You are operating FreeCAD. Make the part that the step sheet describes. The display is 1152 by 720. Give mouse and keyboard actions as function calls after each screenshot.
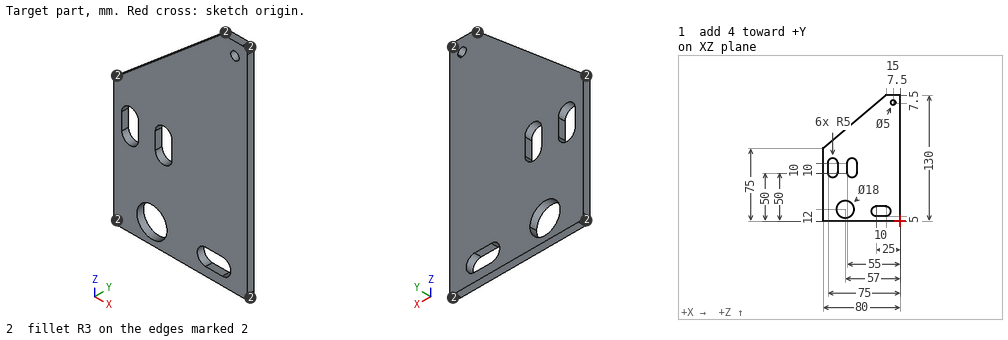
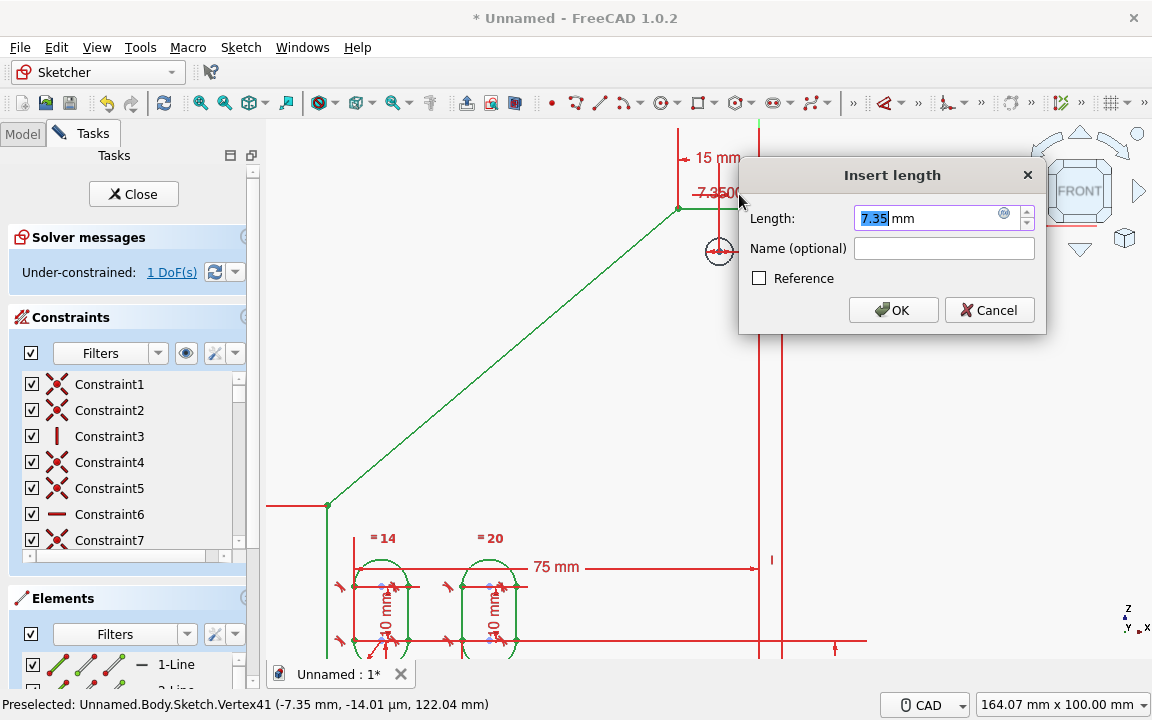
text(7.5)
key(Return)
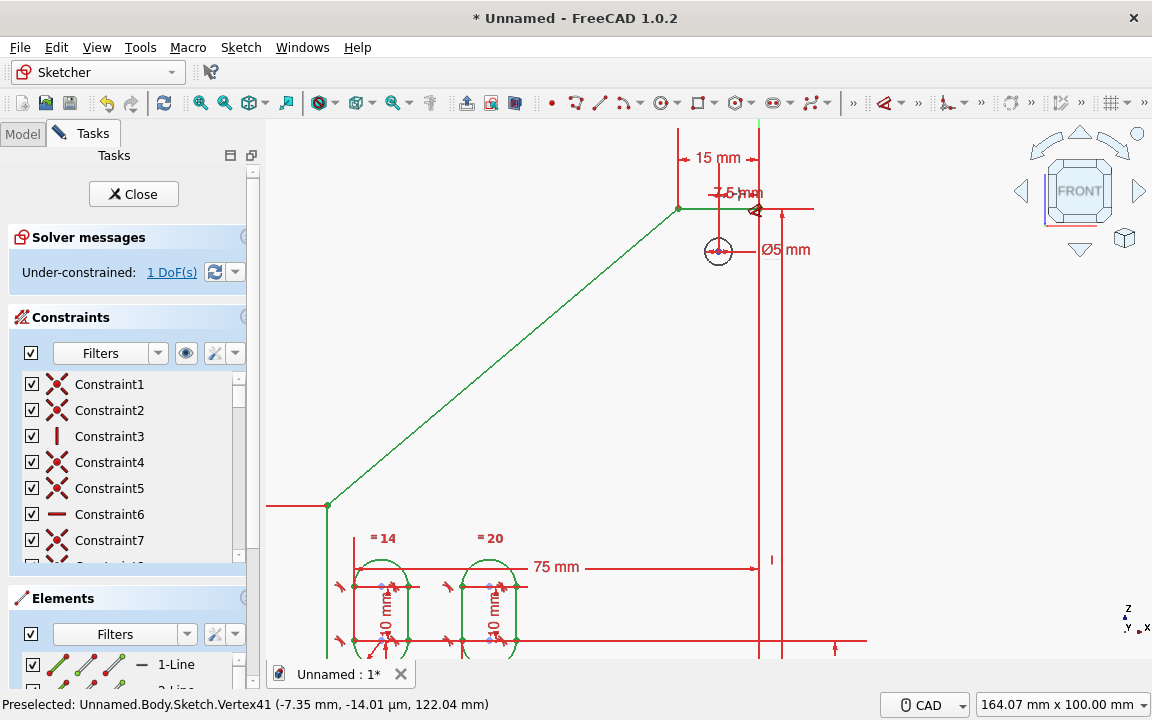
click(678, 209)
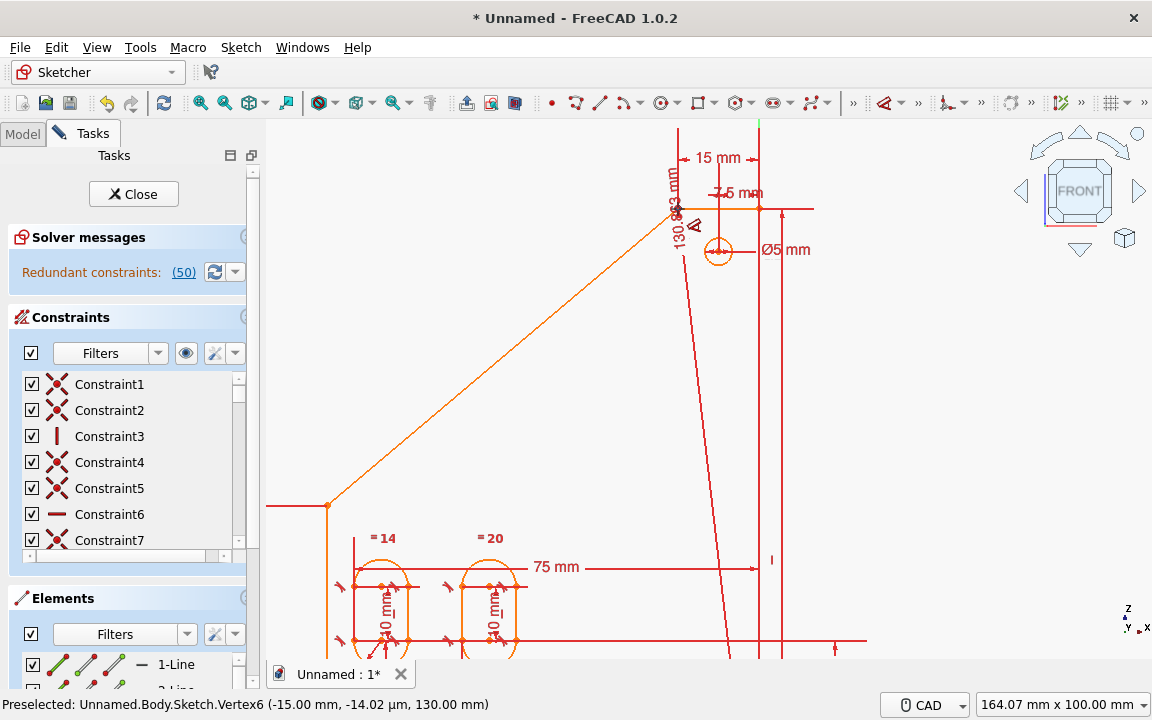
click(719, 252)
click(644, 220)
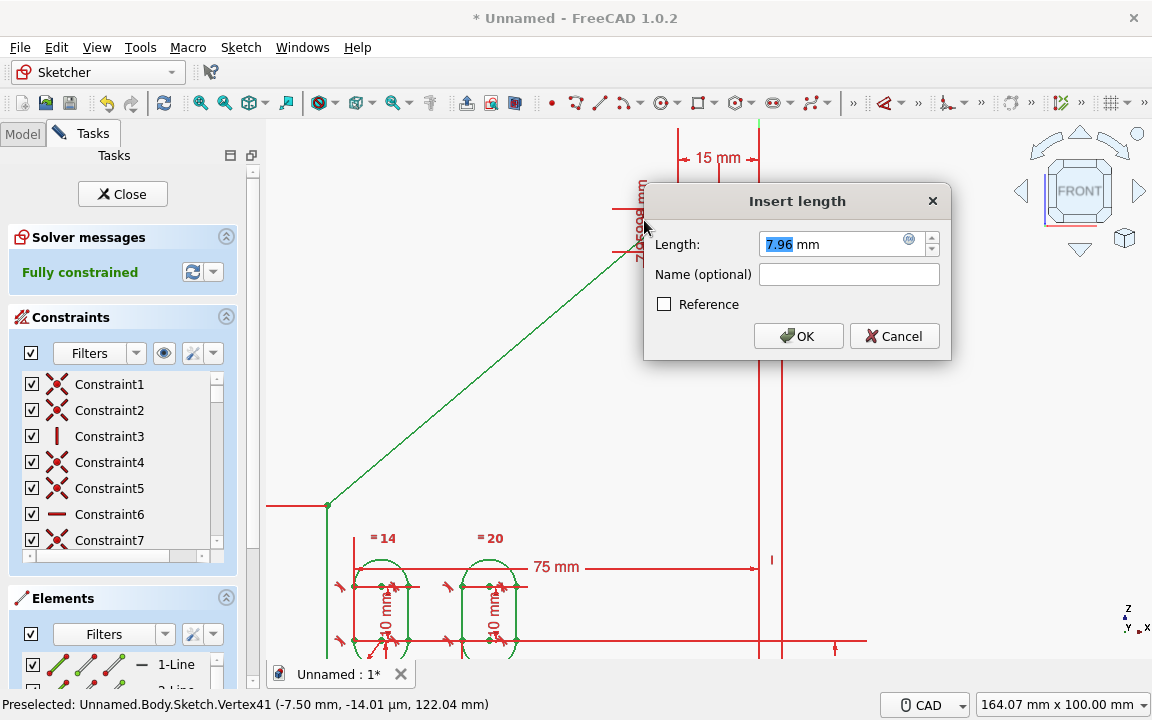
text(7.5)
key(Return)
key(Escape)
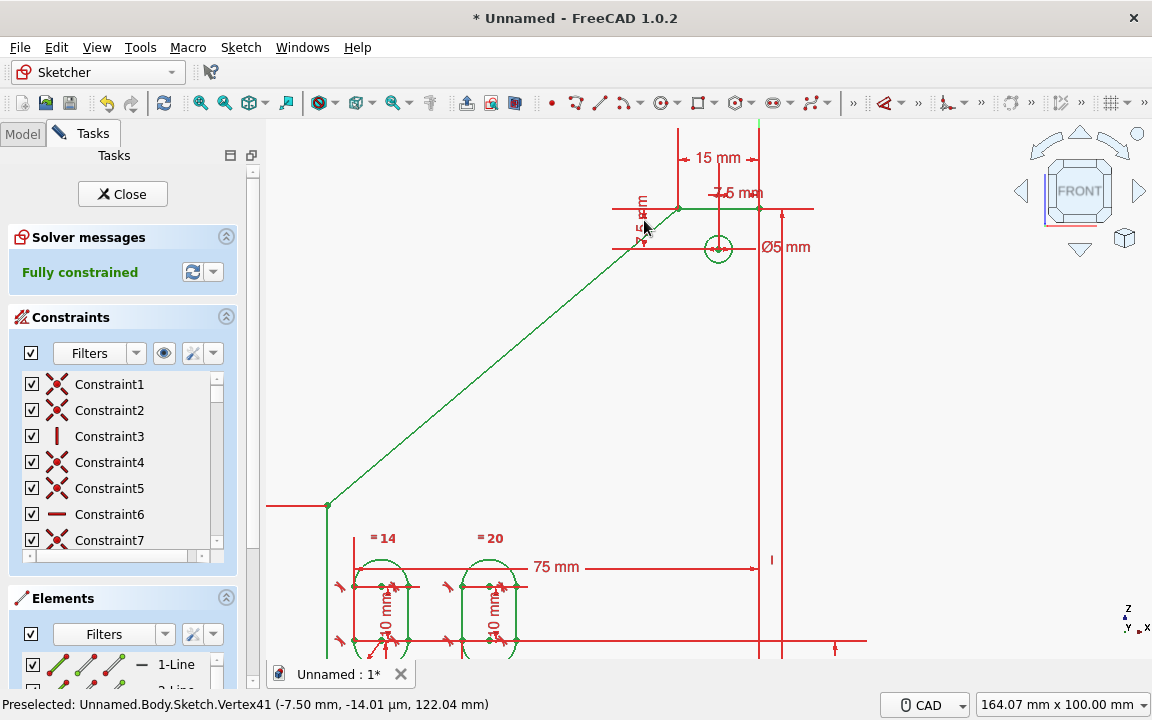
click(123, 194)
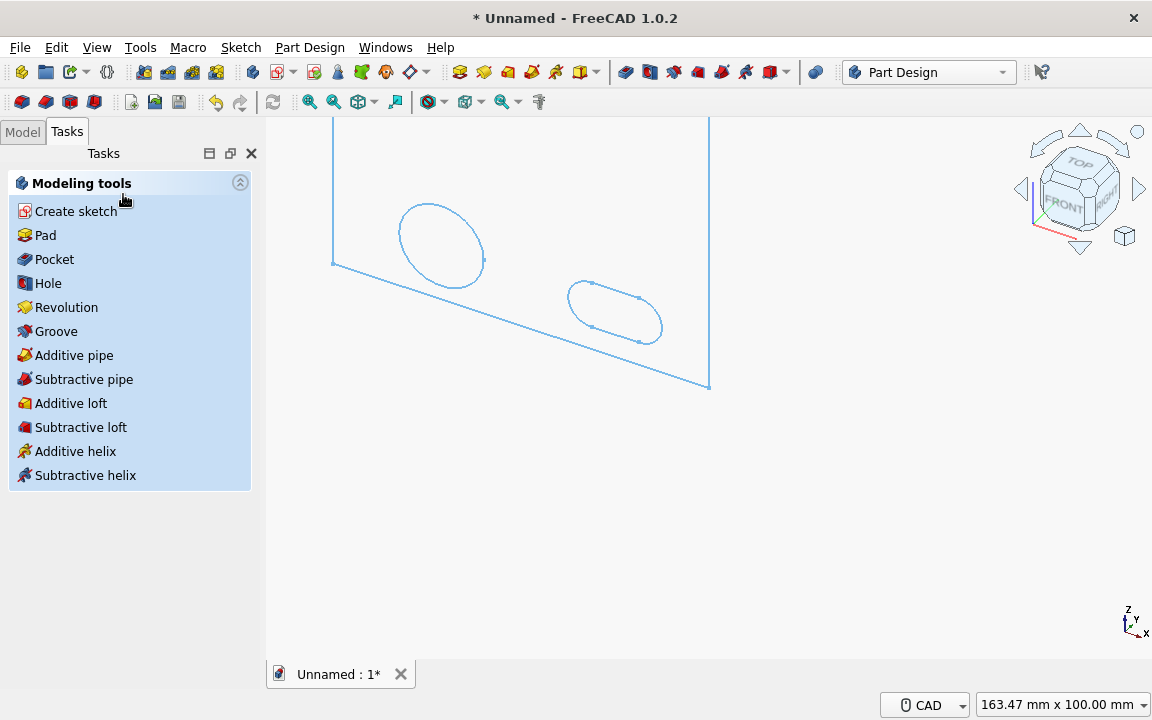
click(460, 72)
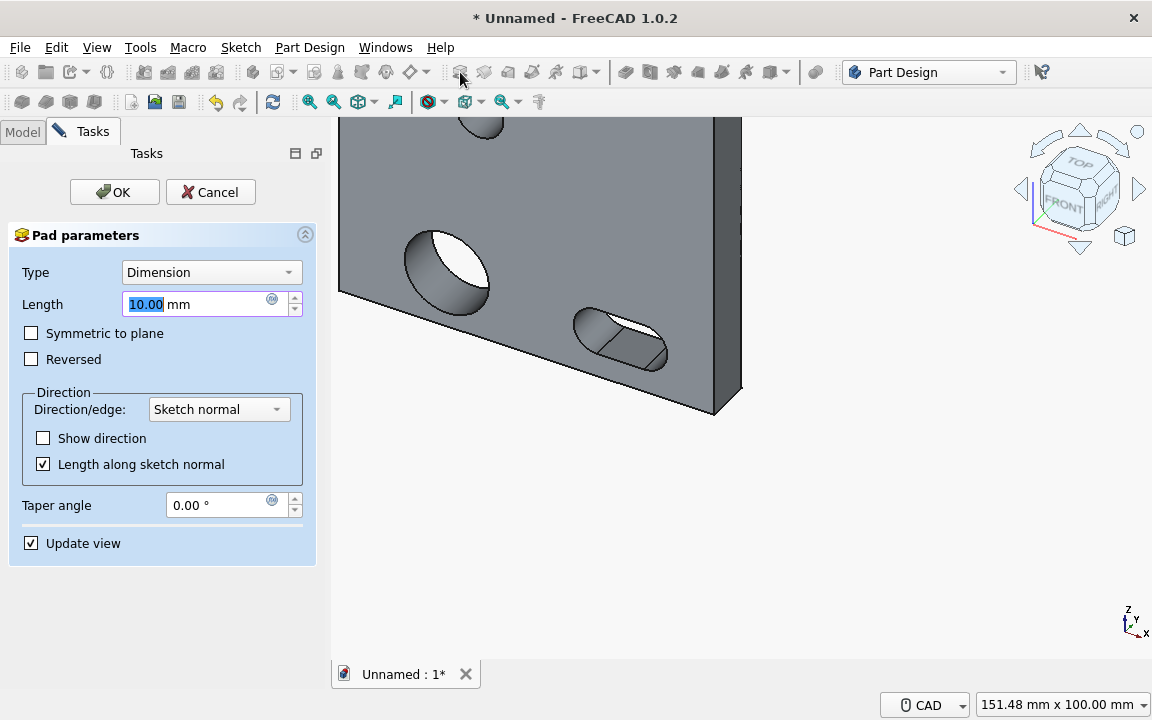
text(4)
key(Tab)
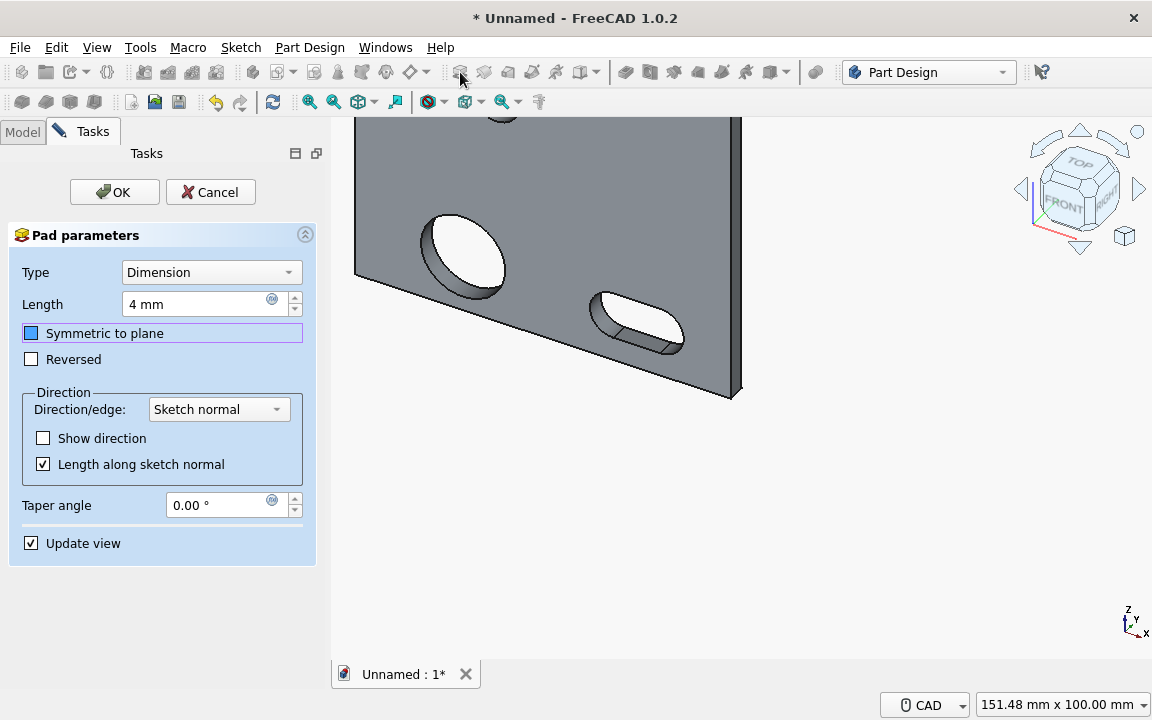
click(30, 359)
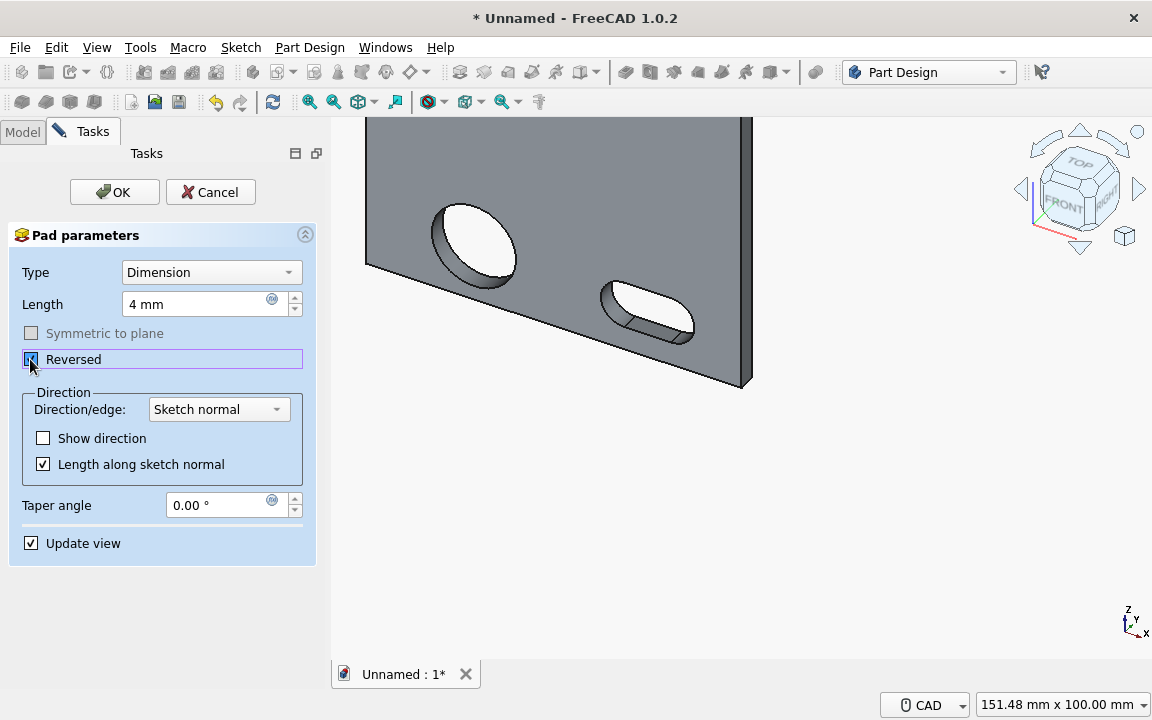
click(115, 192)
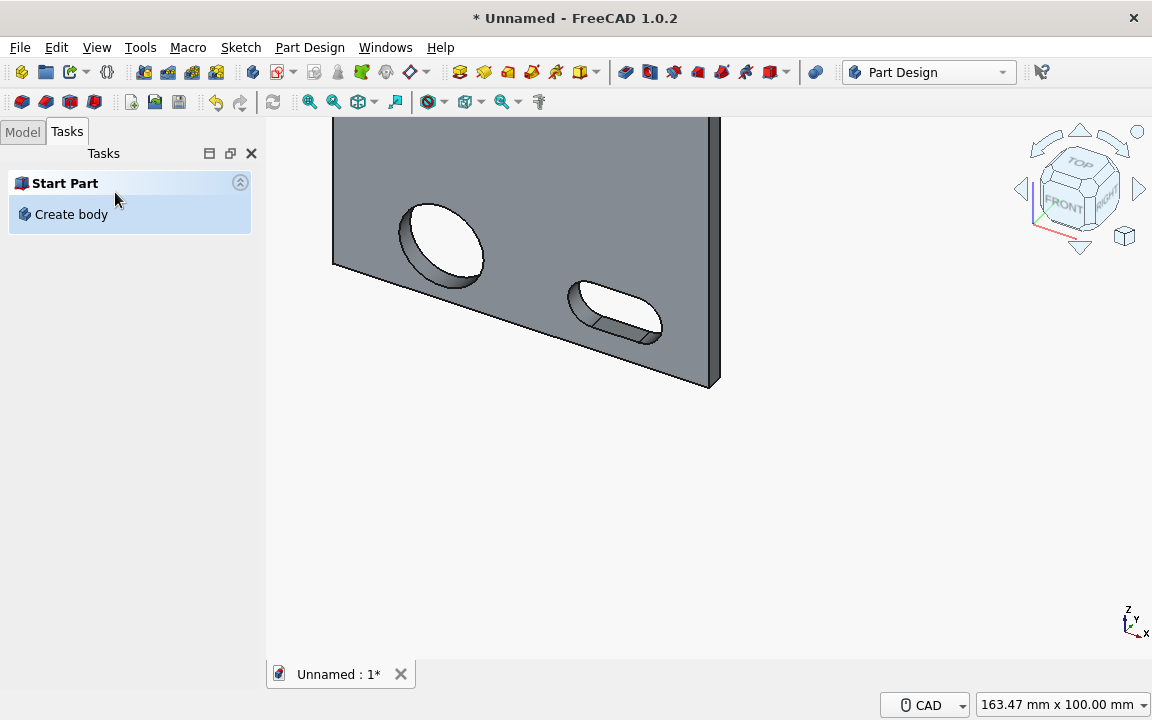
click(310, 102)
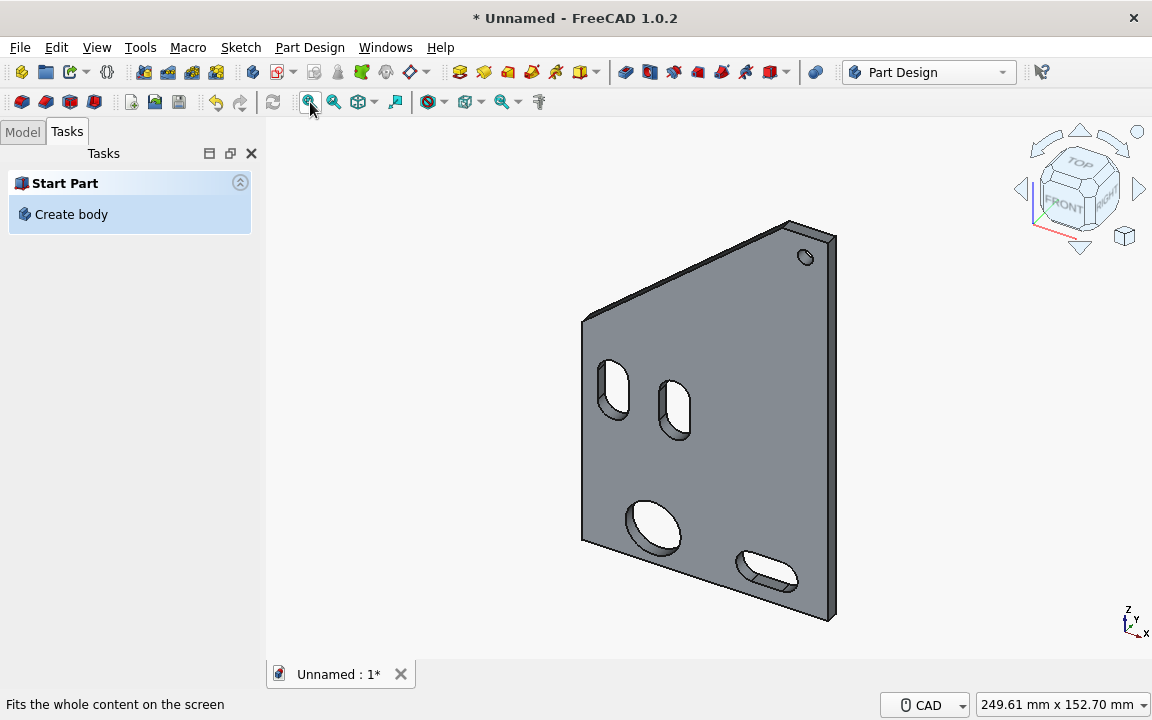
click(833, 237)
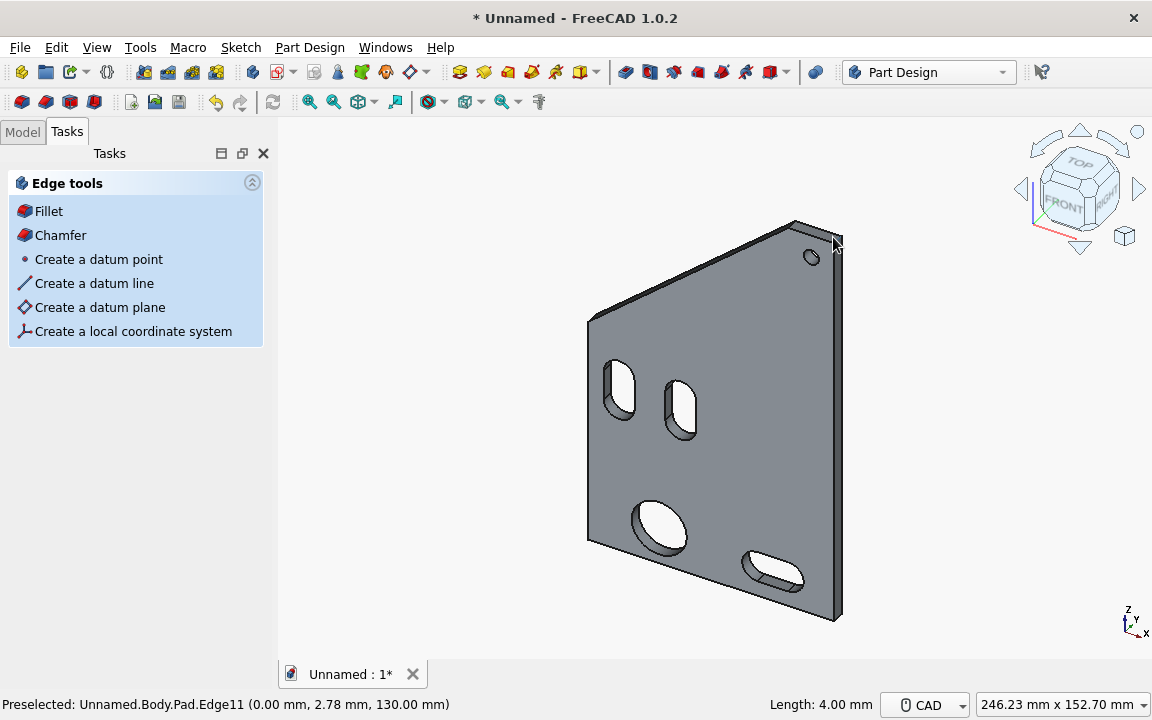
scroll(792, 223, up, 6)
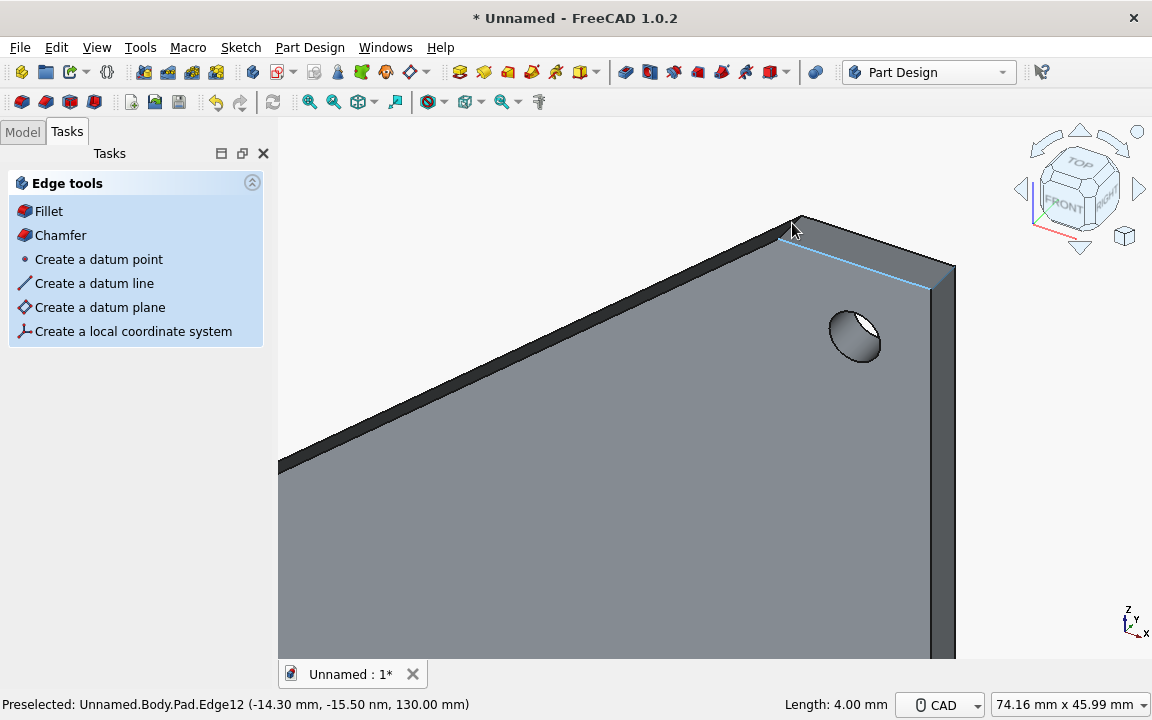
click(310, 102)